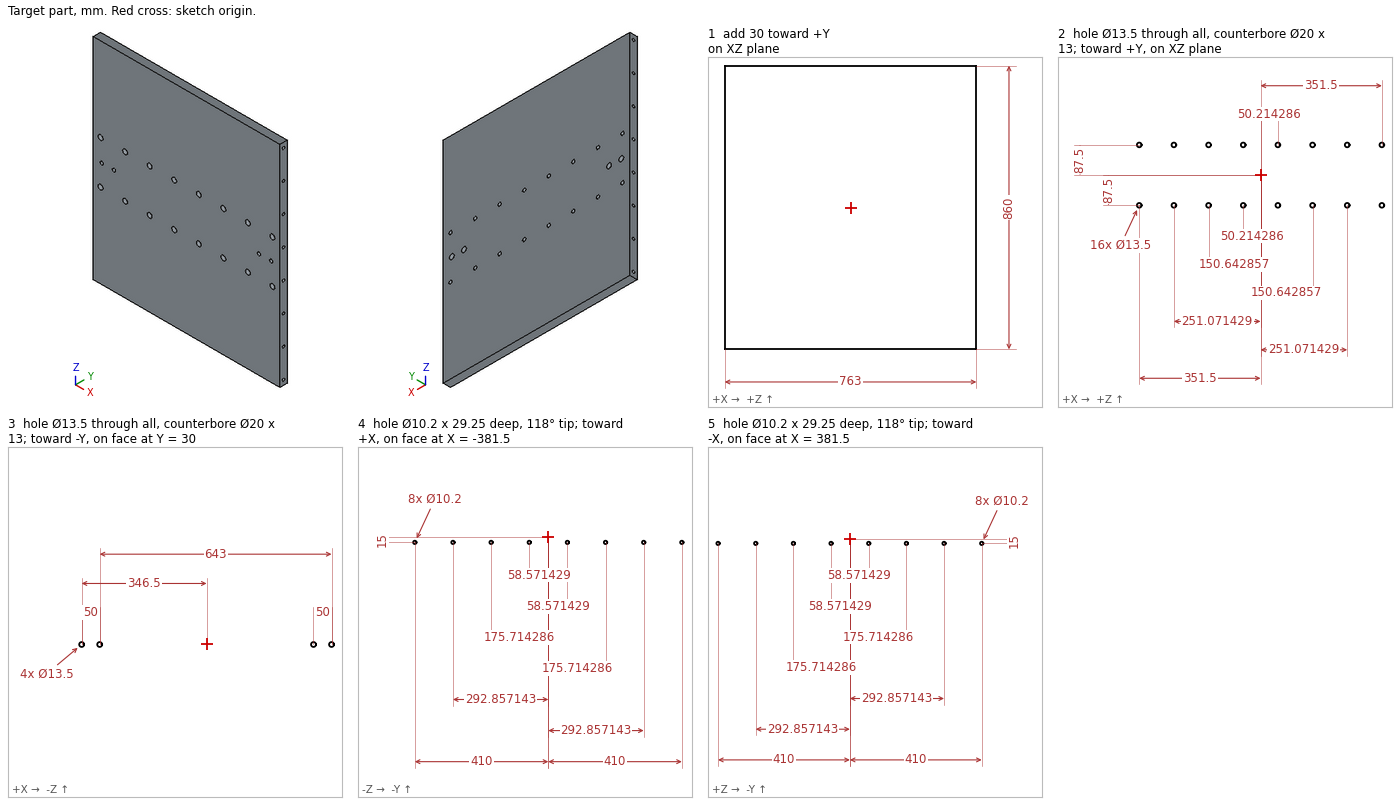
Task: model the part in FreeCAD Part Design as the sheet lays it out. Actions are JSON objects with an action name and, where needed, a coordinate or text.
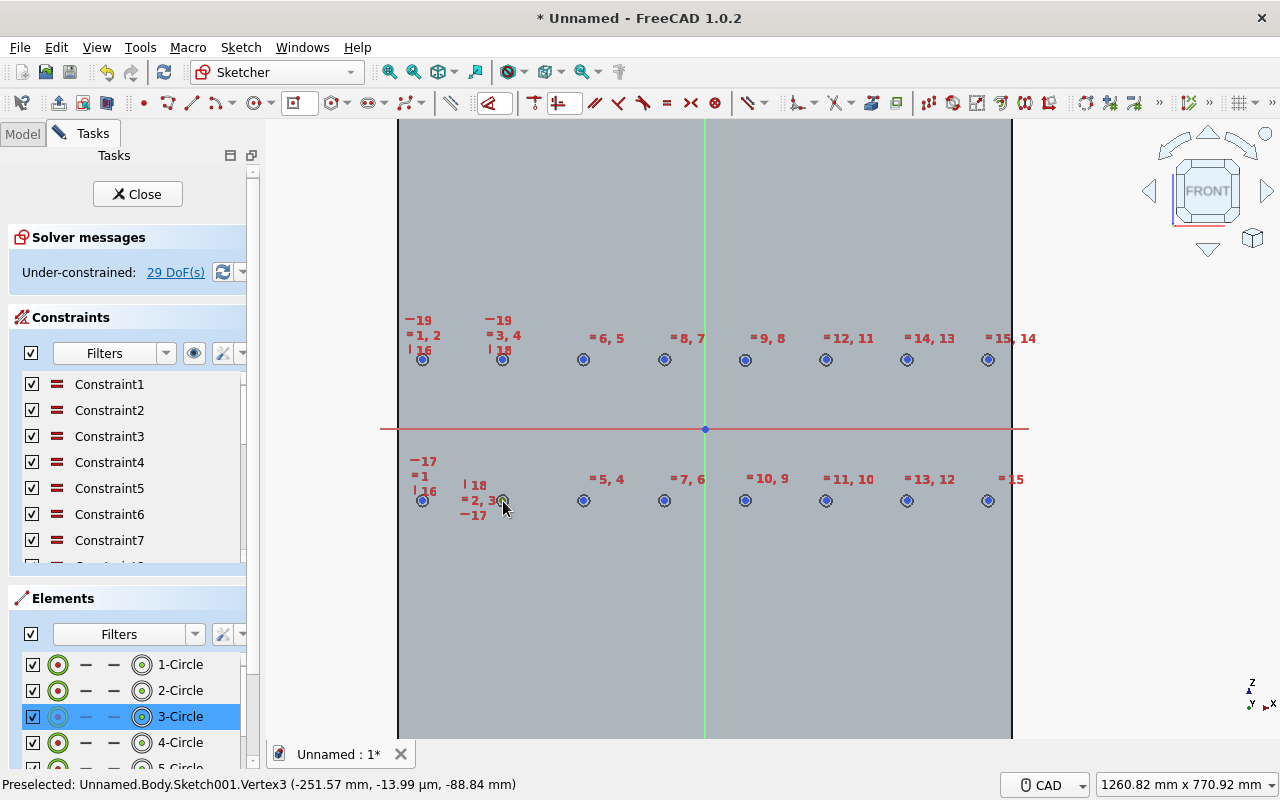
{"action": "left_click", "coordinate": [584, 501]}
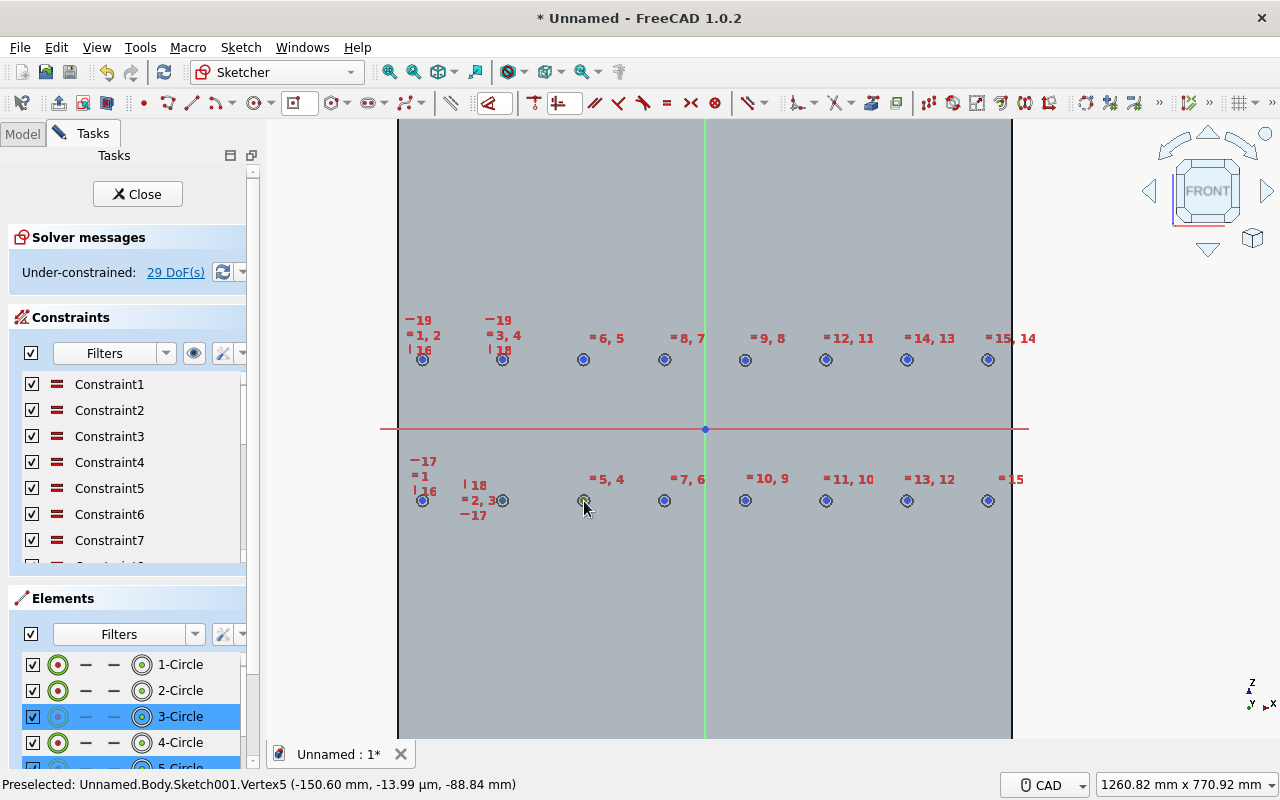
{"action": "key", "text": "h"}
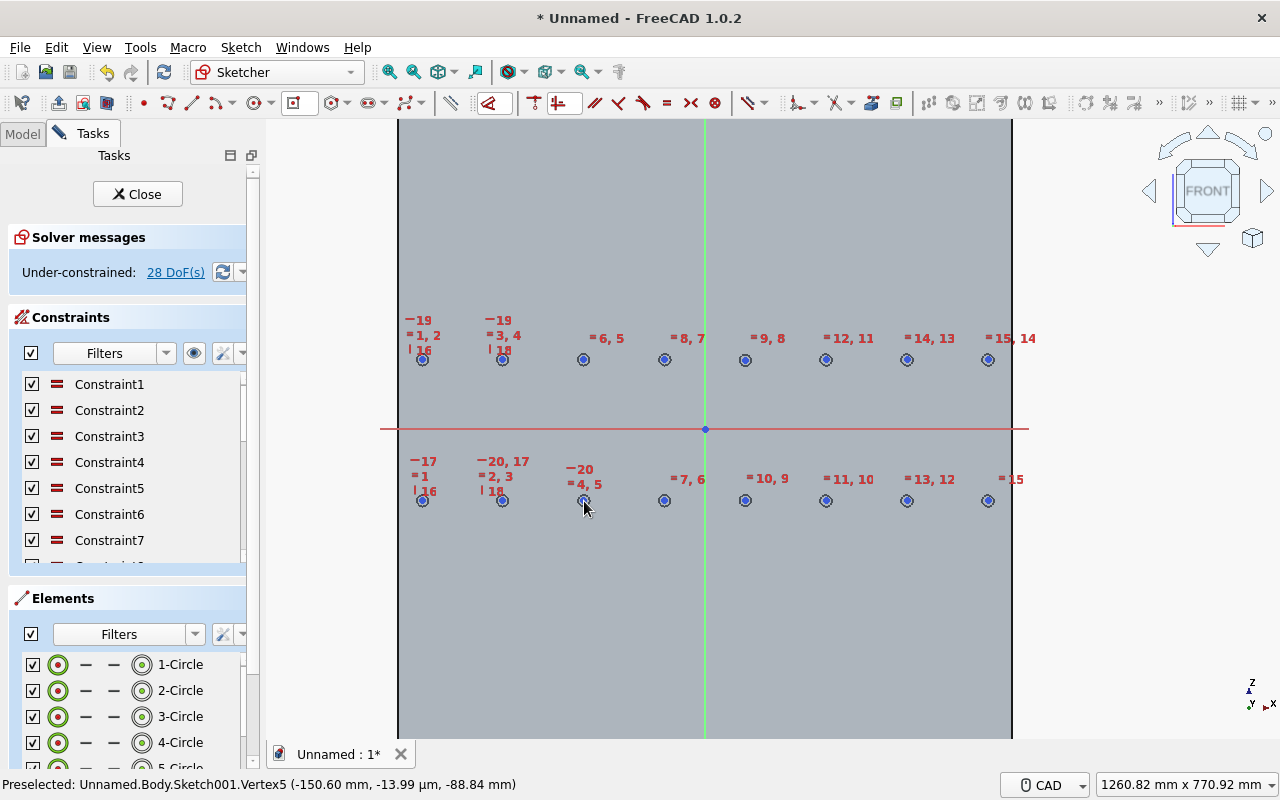
{"action": "left_click", "coordinate": [584, 501]}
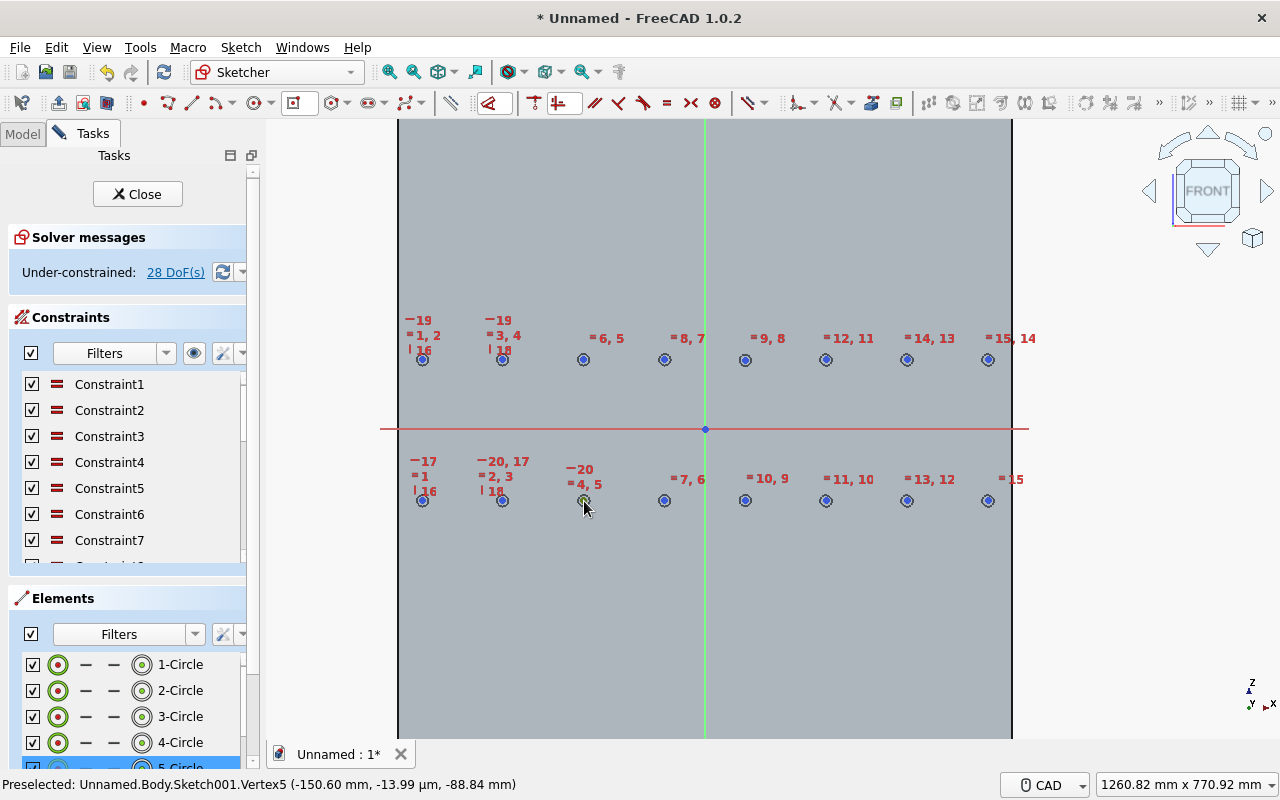
{"action": "left_click", "coordinate": [584, 360]}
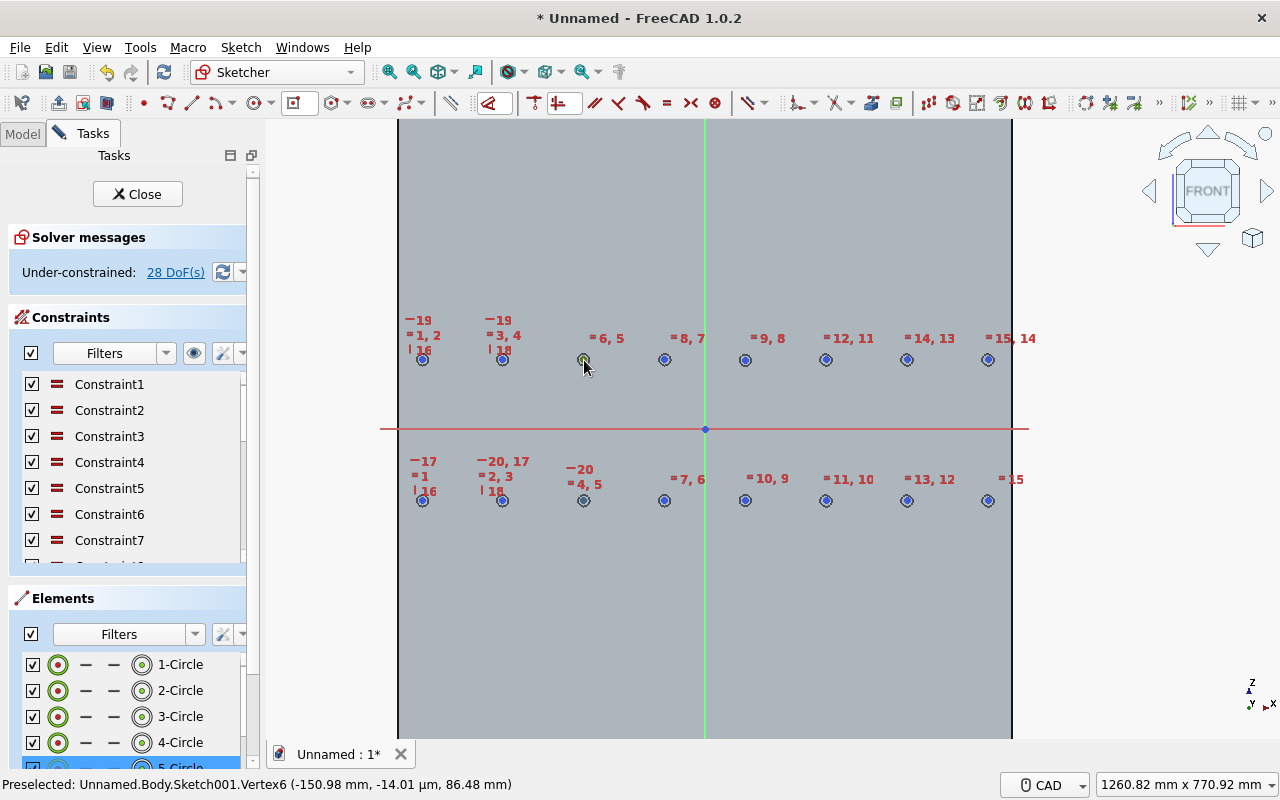
{"action": "left_click", "coordinate": [576, 104]}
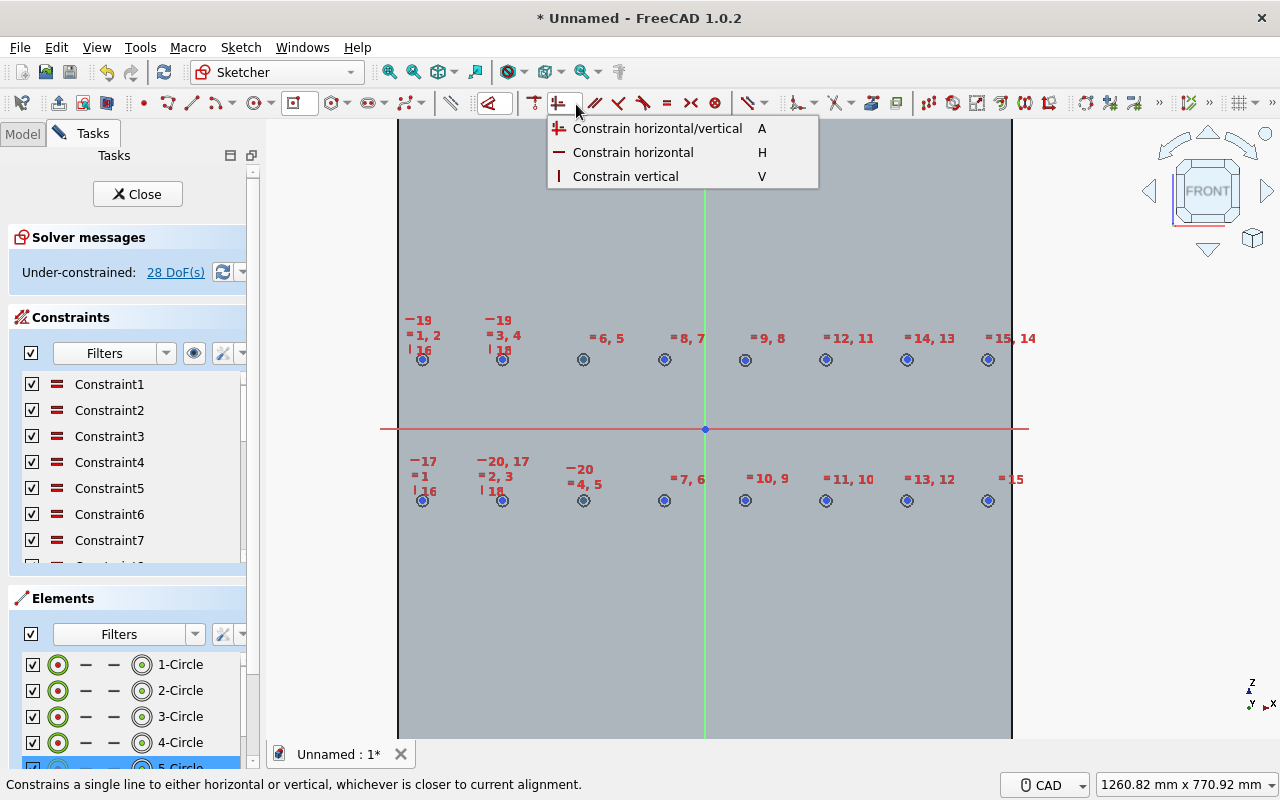
{"action": "left_click", "coordinate": [683, 176]}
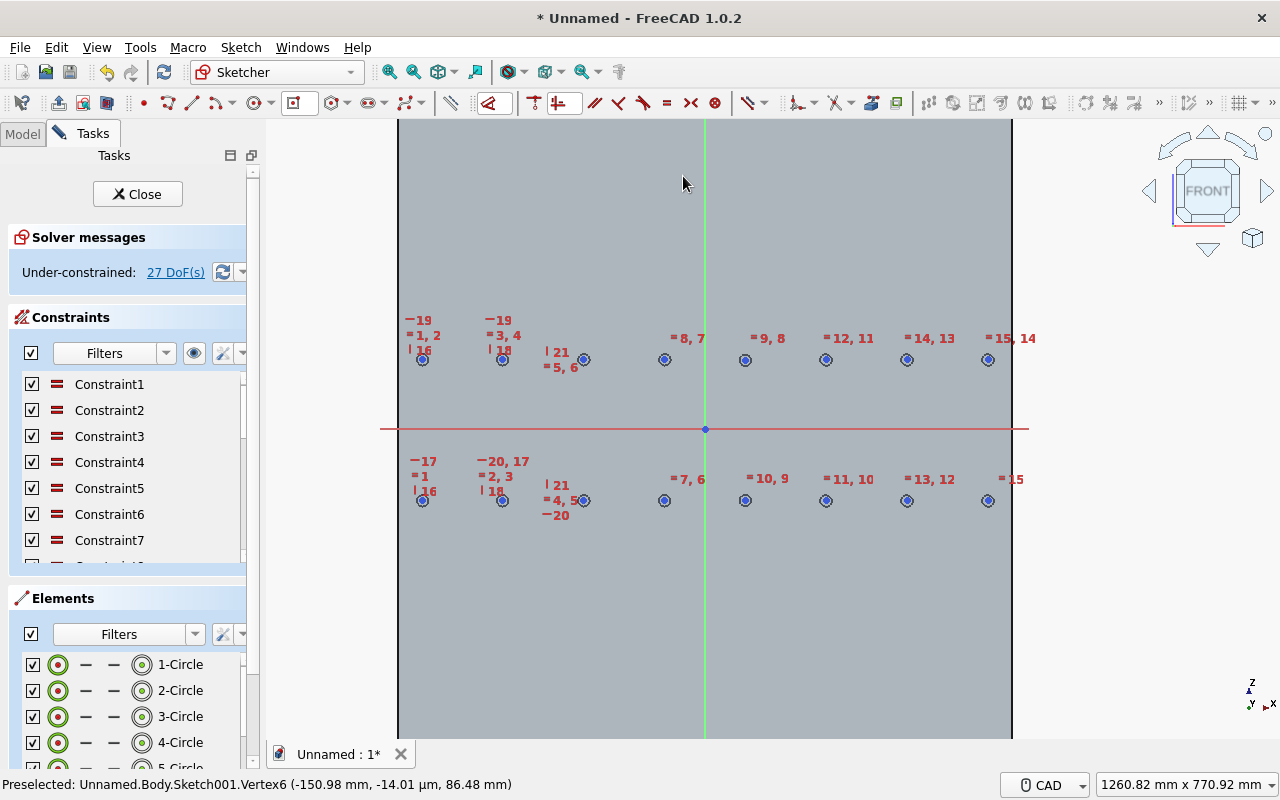
{"action": "left_click", "coordinate": [503, 360]}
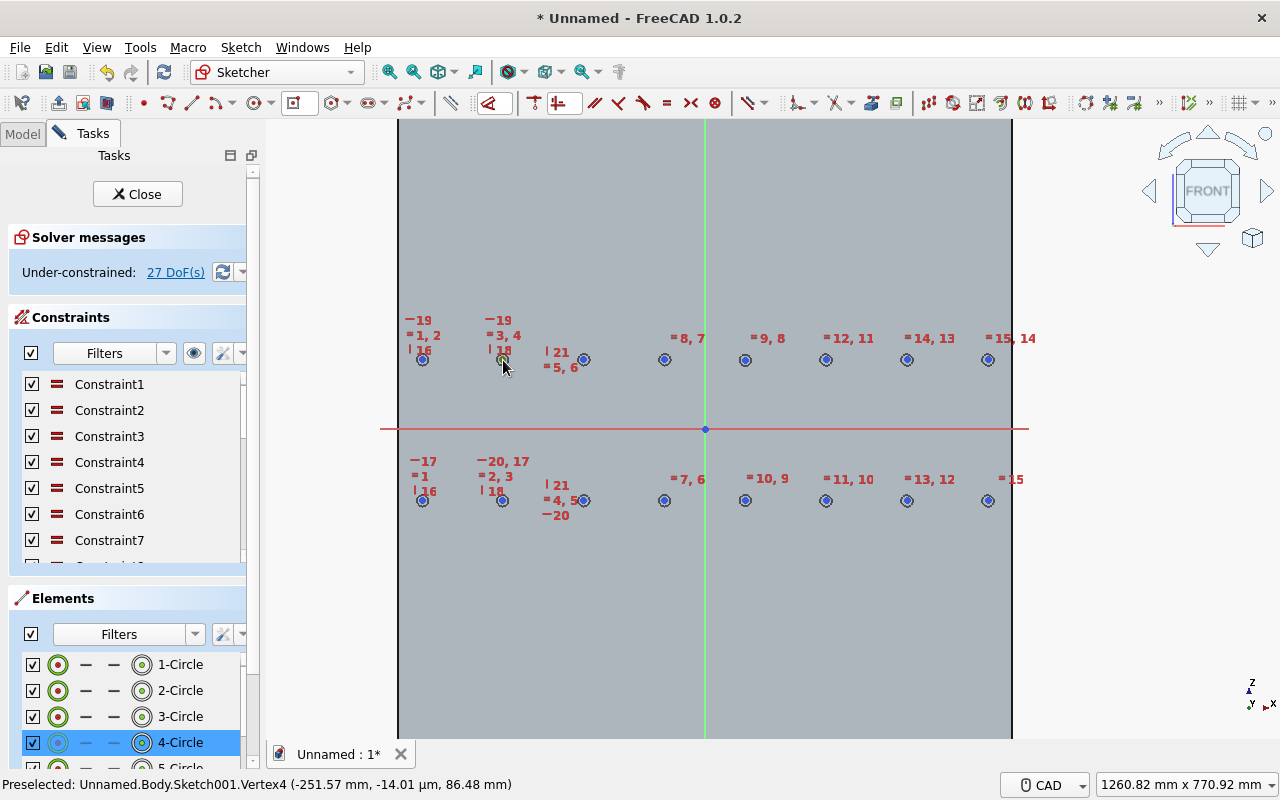
{"action": "left_click", "coordinate": [584, 360]}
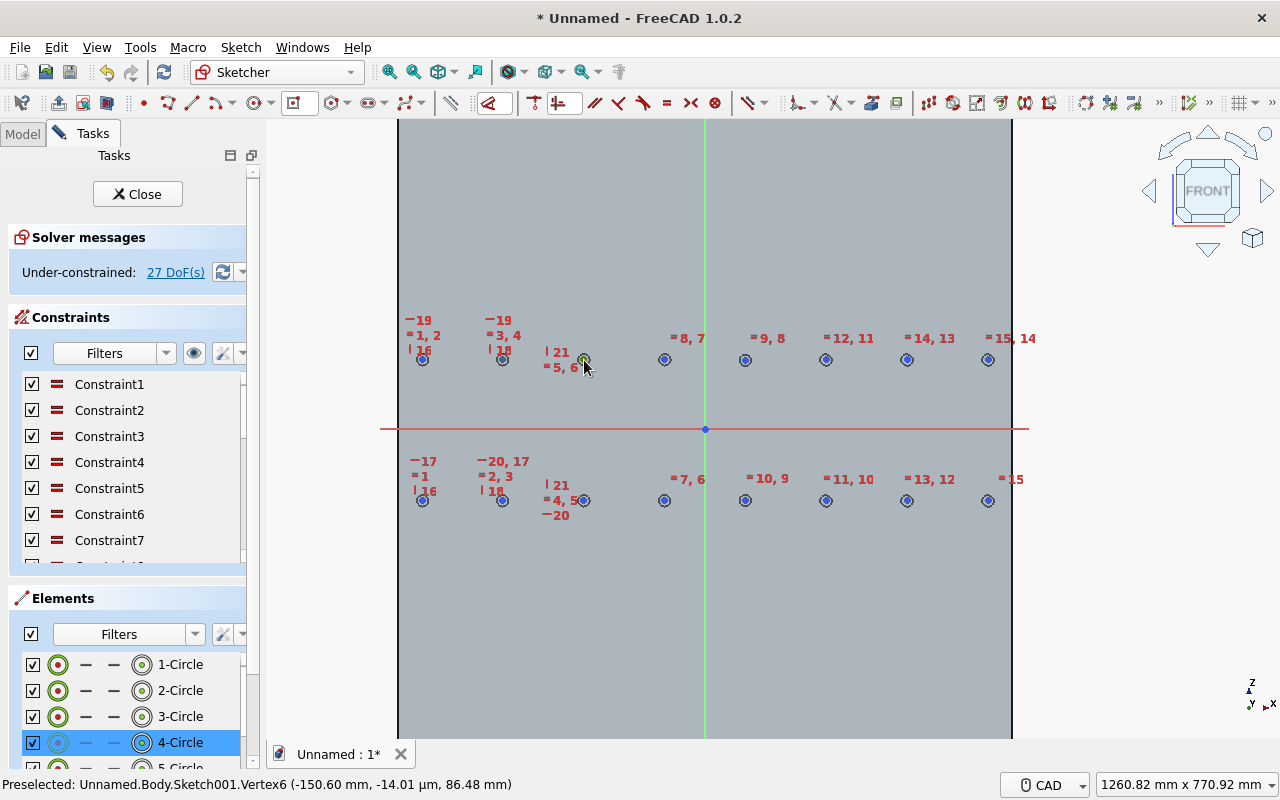
{"action": "key", "text": "h"}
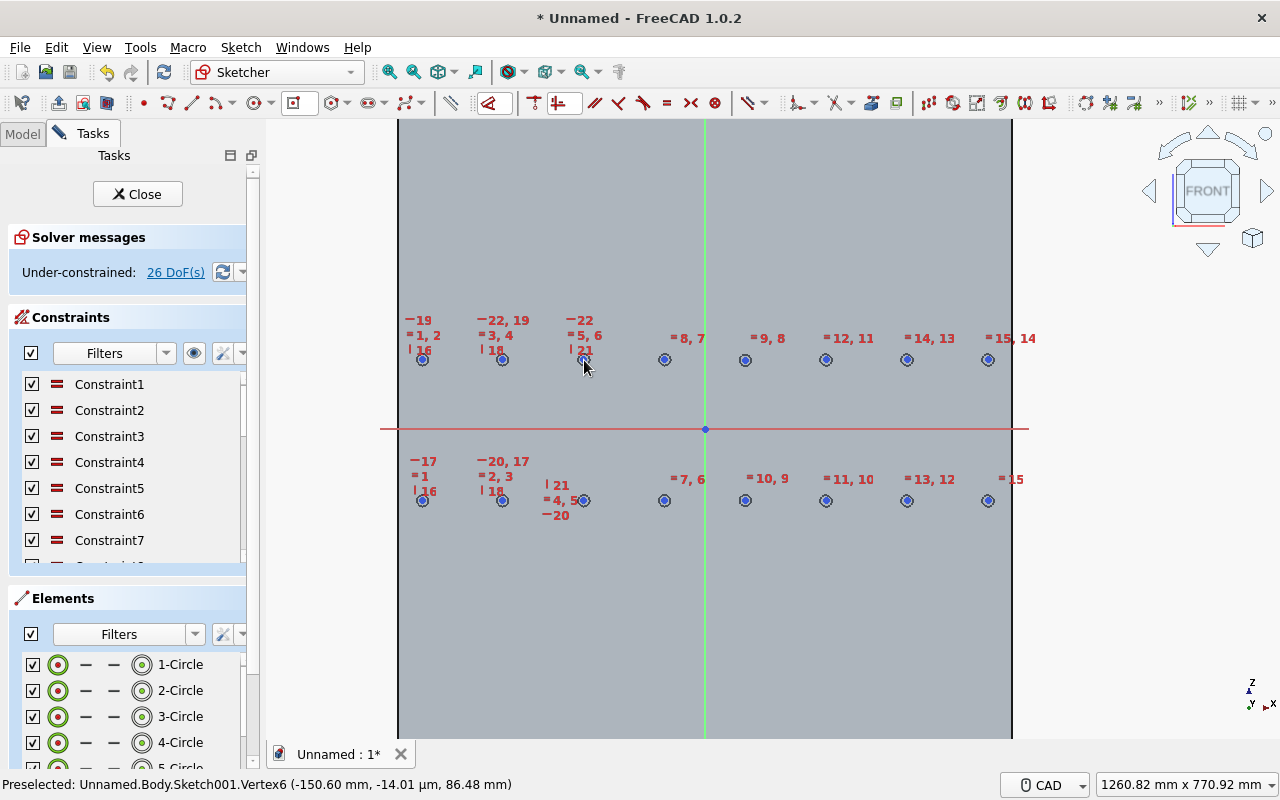
{"action": "left_click", "coordinate": [584, 501]}